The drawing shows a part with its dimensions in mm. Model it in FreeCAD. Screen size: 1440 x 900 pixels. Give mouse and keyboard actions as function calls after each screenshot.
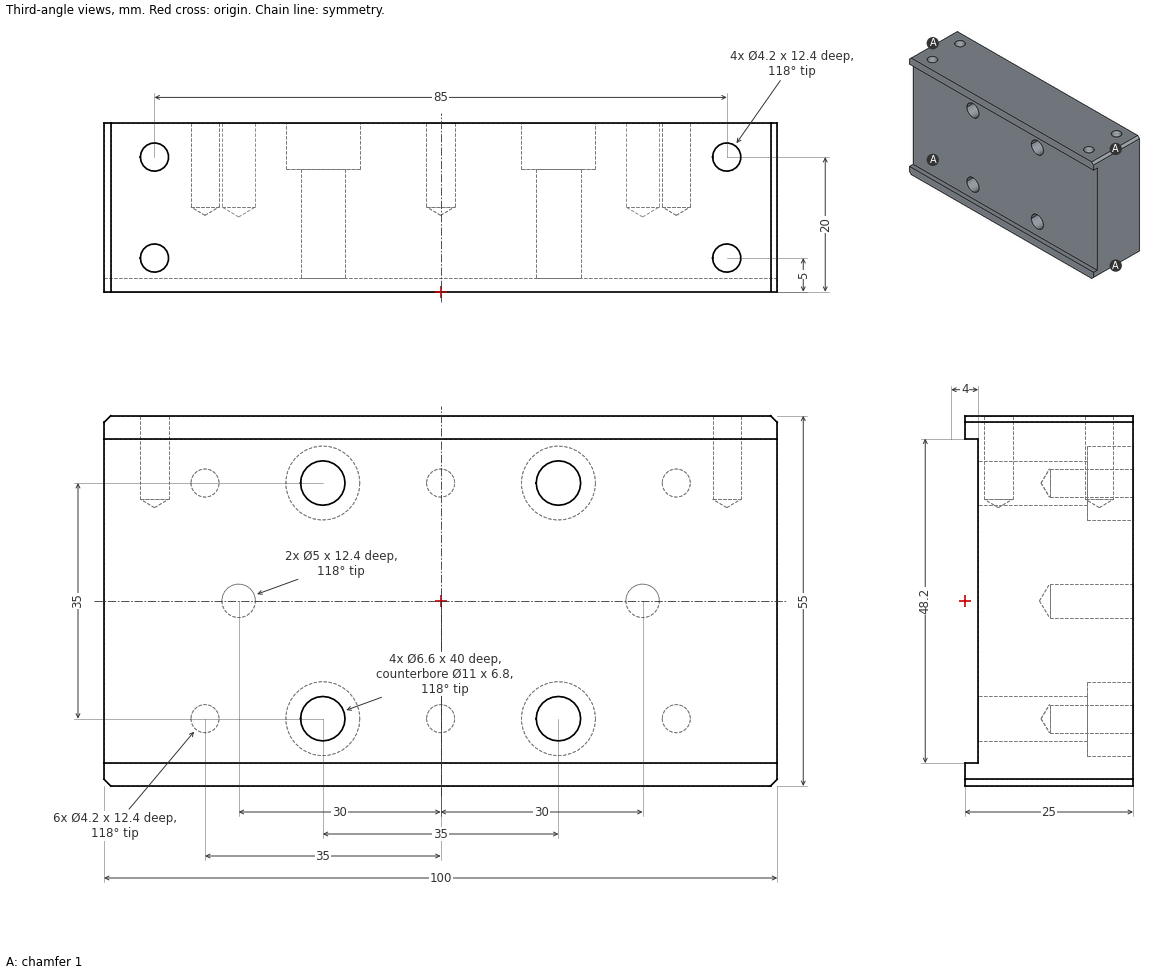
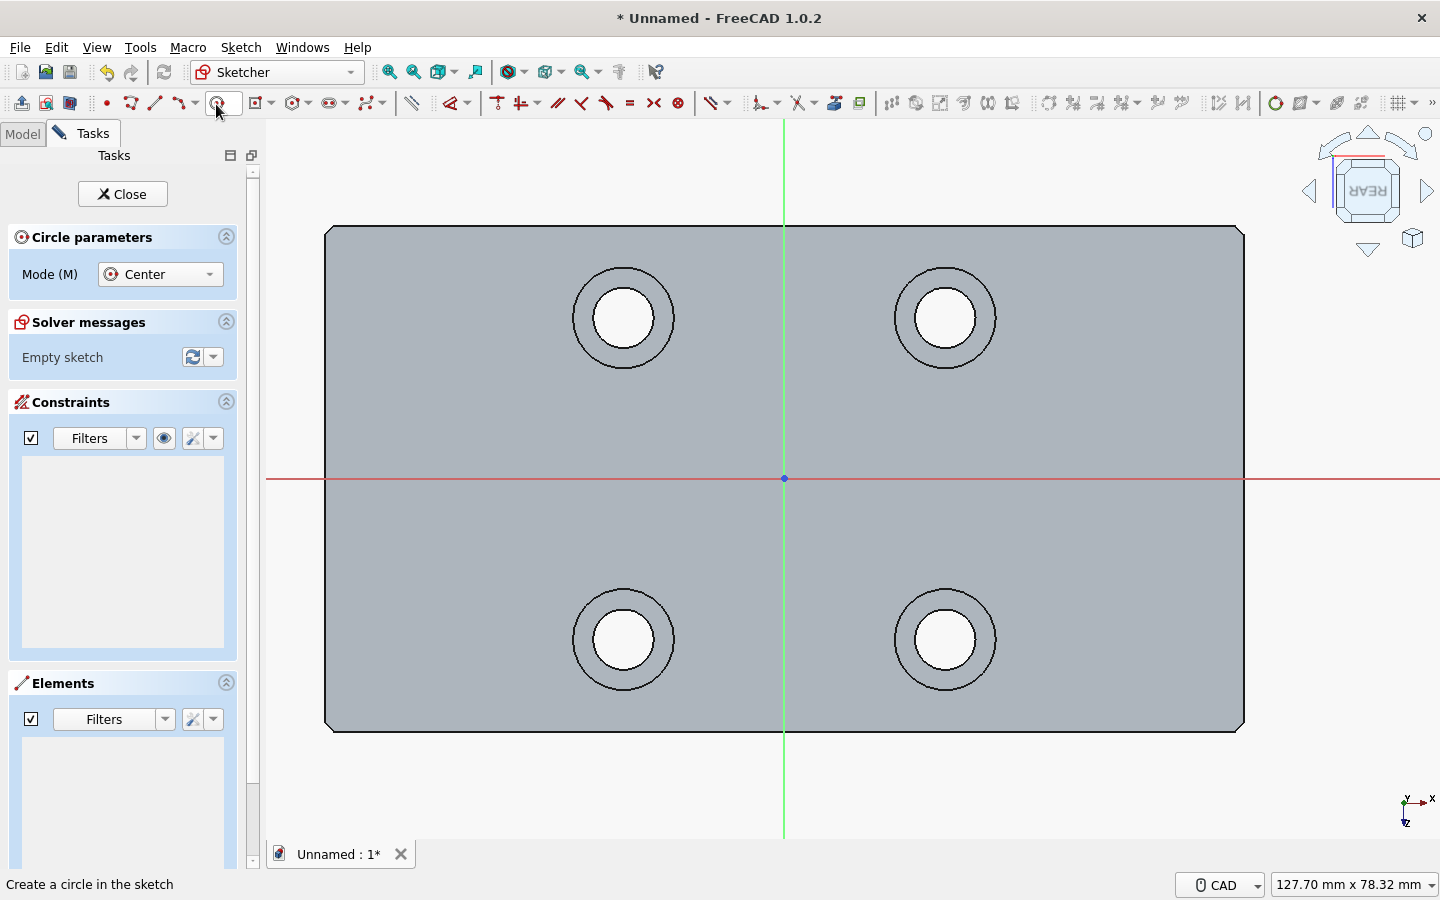
click(463, 318)
move(476, 304)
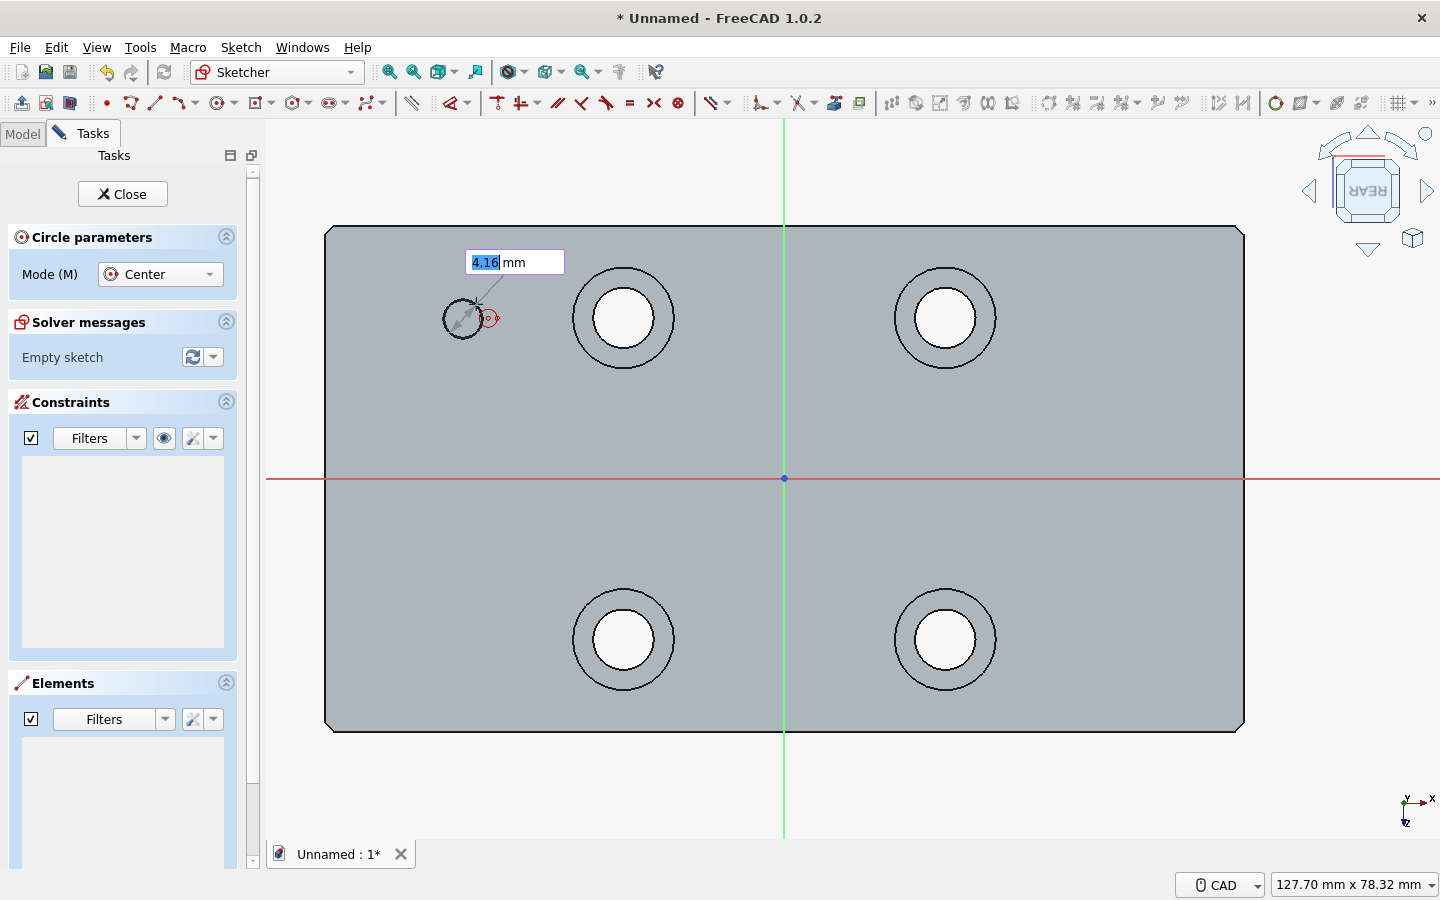
text(4.2)
key(Return)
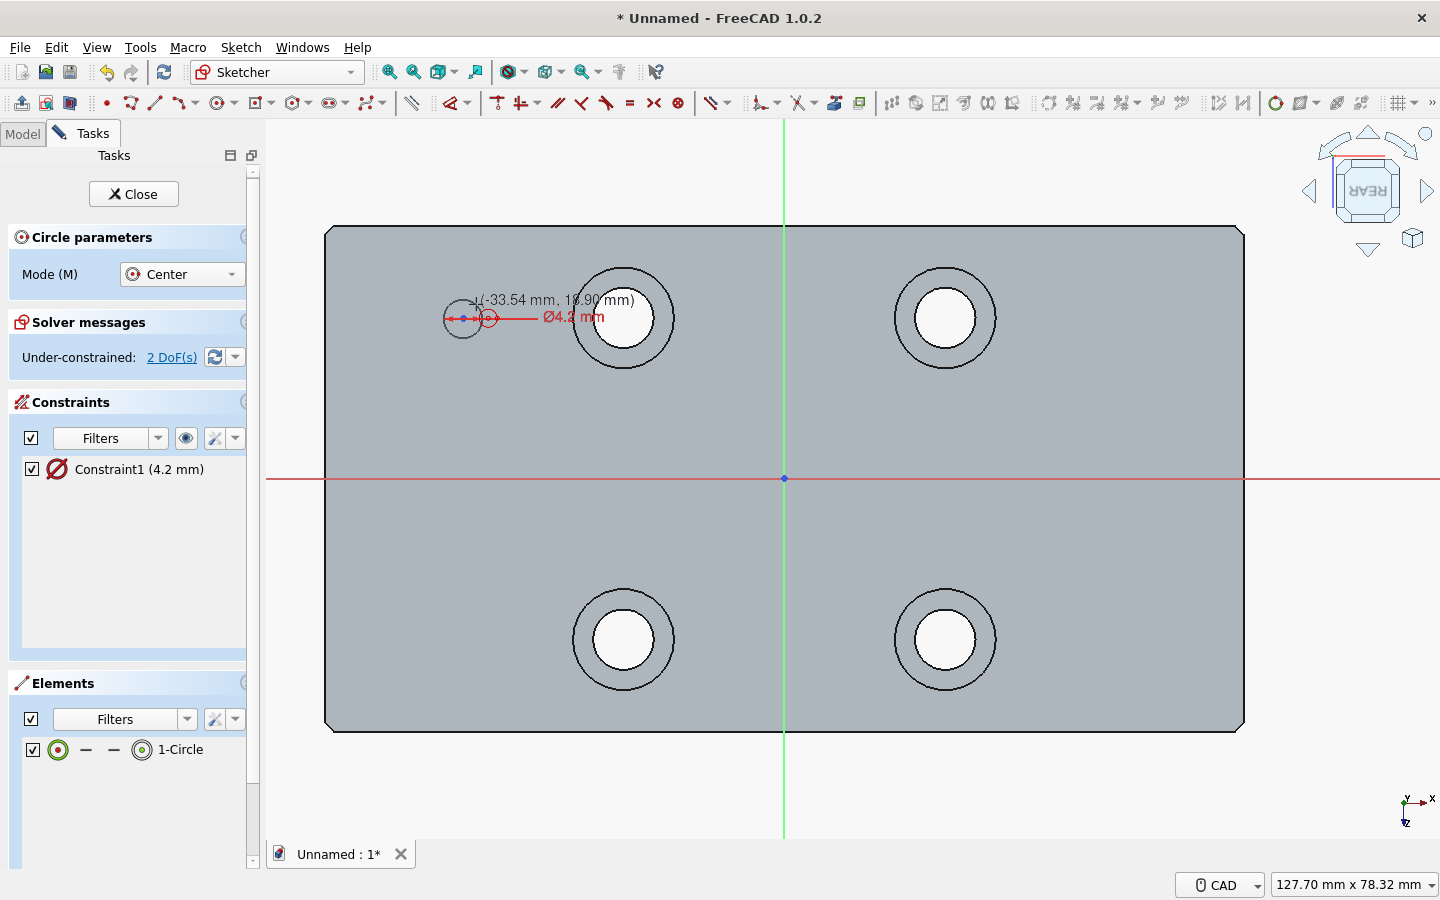
click(463, 640)
move(476, 626)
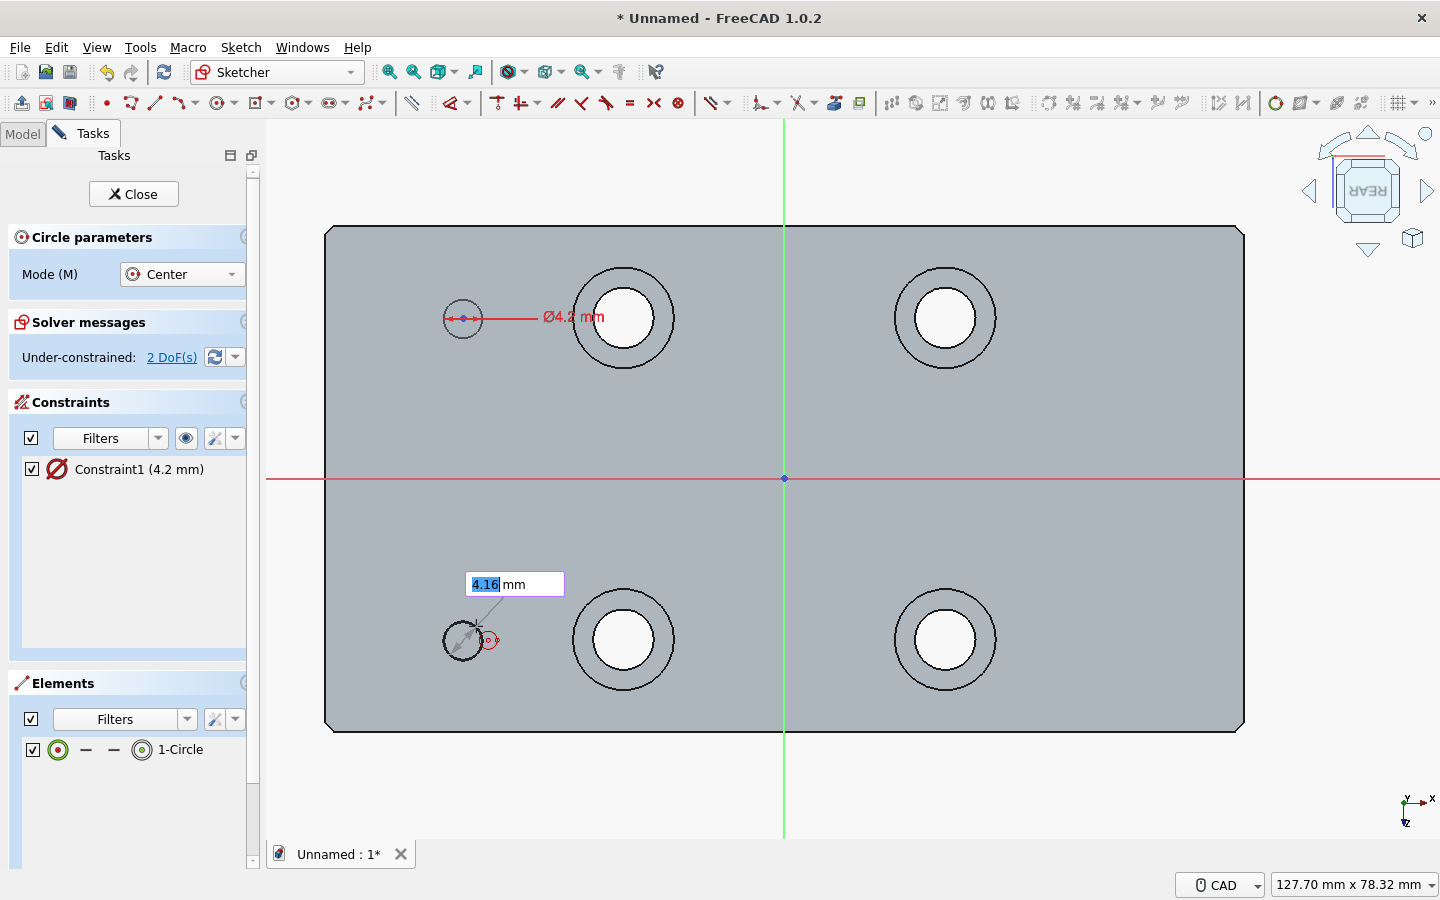
text(4.2)
key(Return)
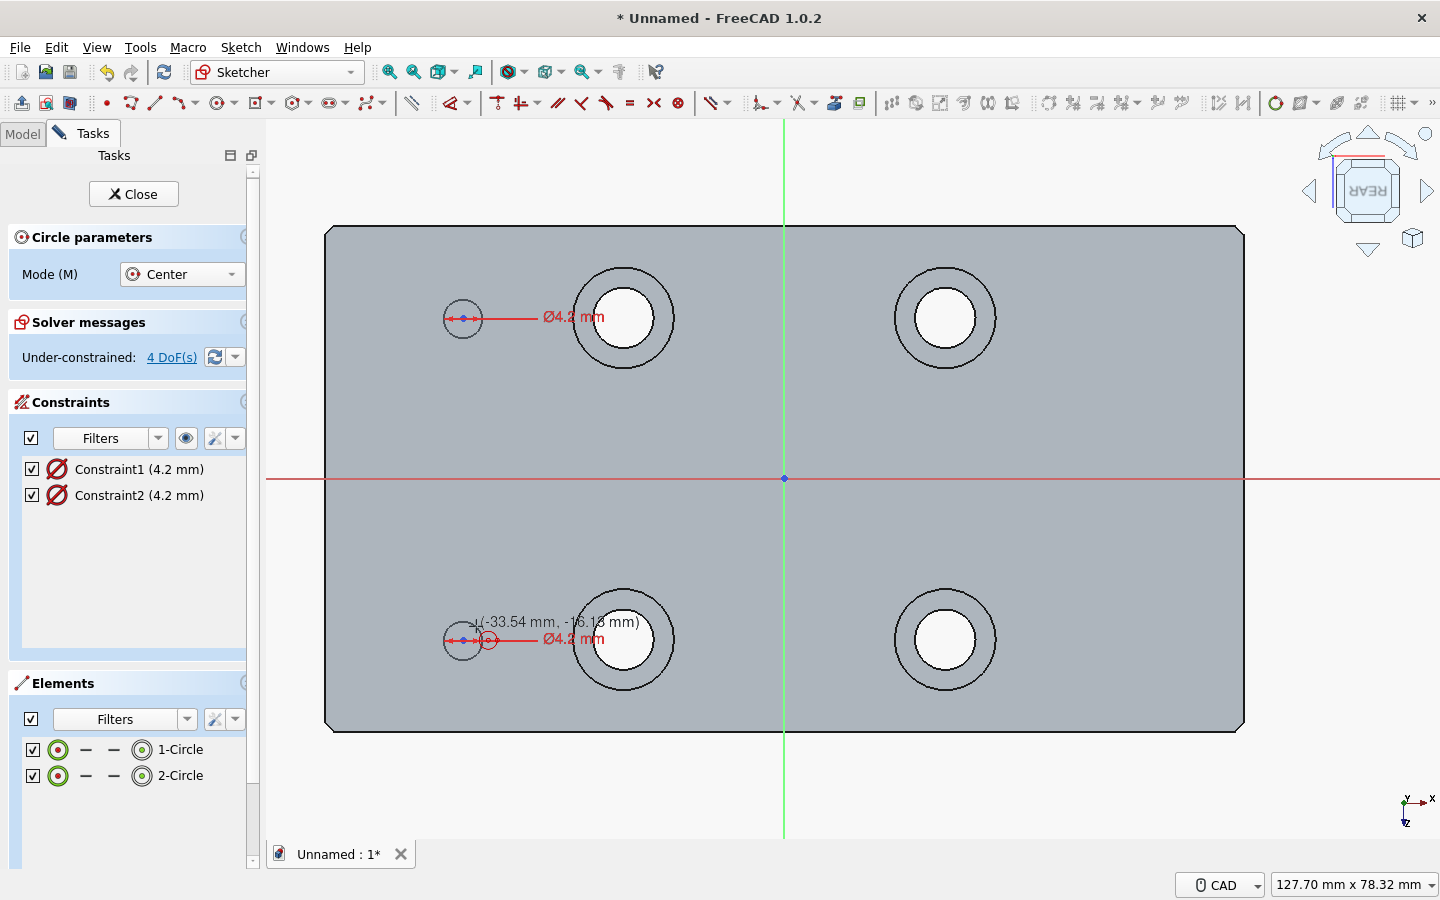
click(1106, 318)
move(1120, 304)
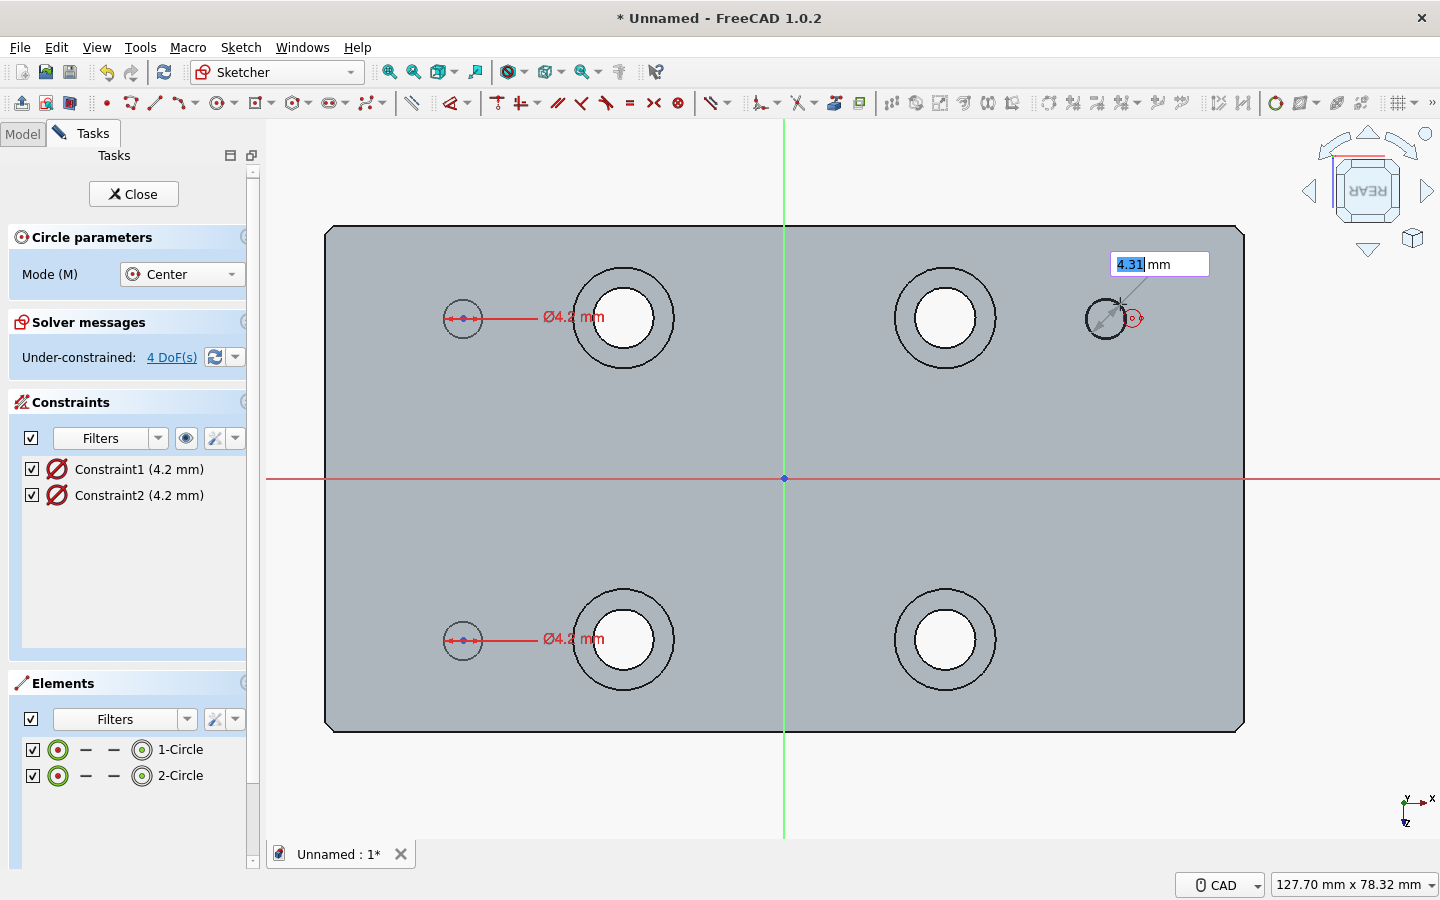
text(4.2)
key(Return)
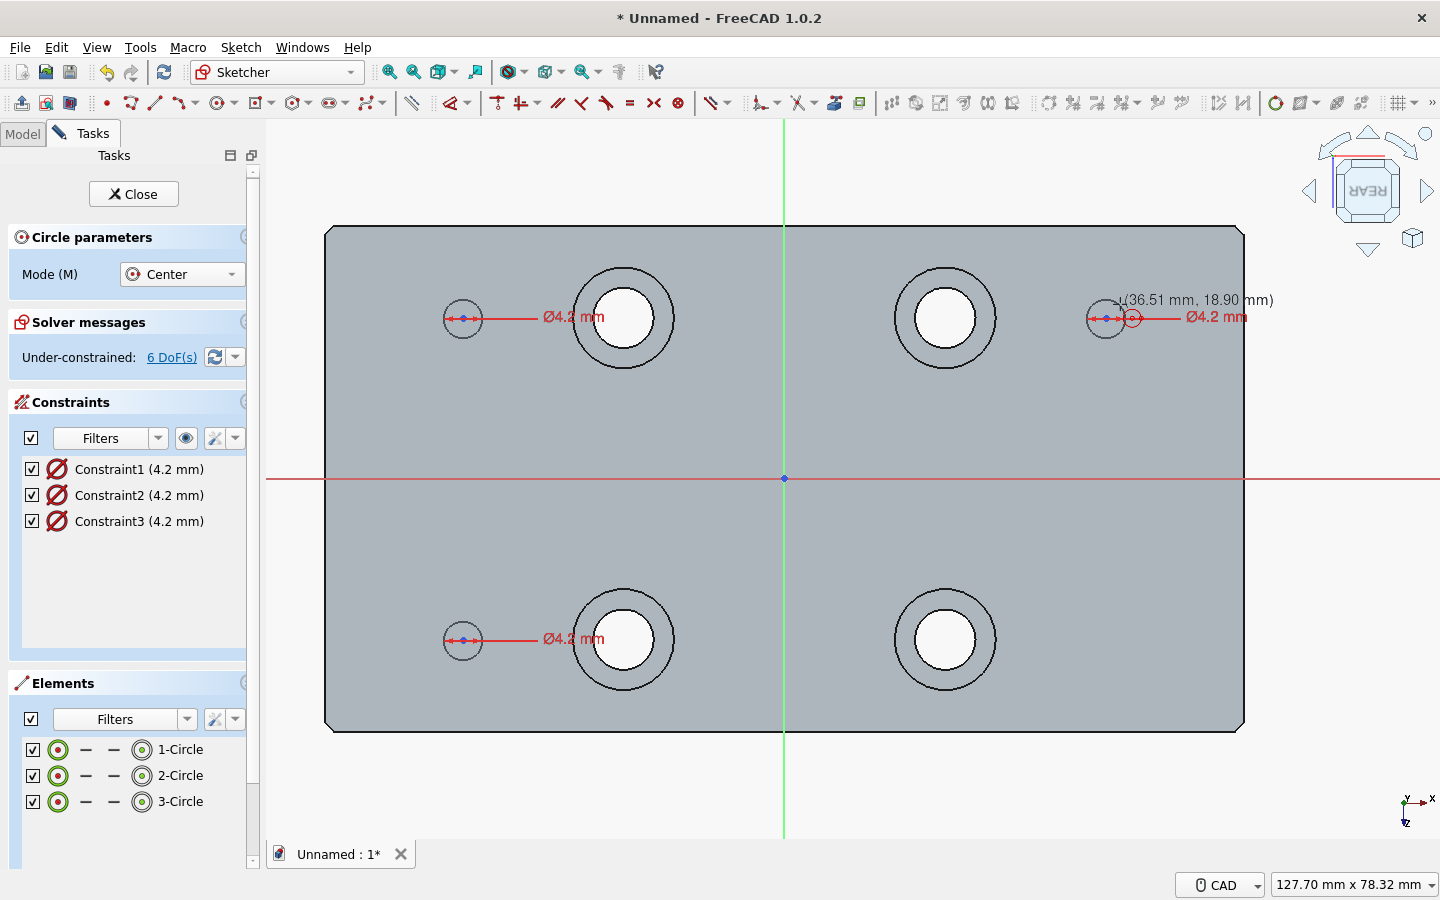
click(1106, 640)
move(1120, 626)